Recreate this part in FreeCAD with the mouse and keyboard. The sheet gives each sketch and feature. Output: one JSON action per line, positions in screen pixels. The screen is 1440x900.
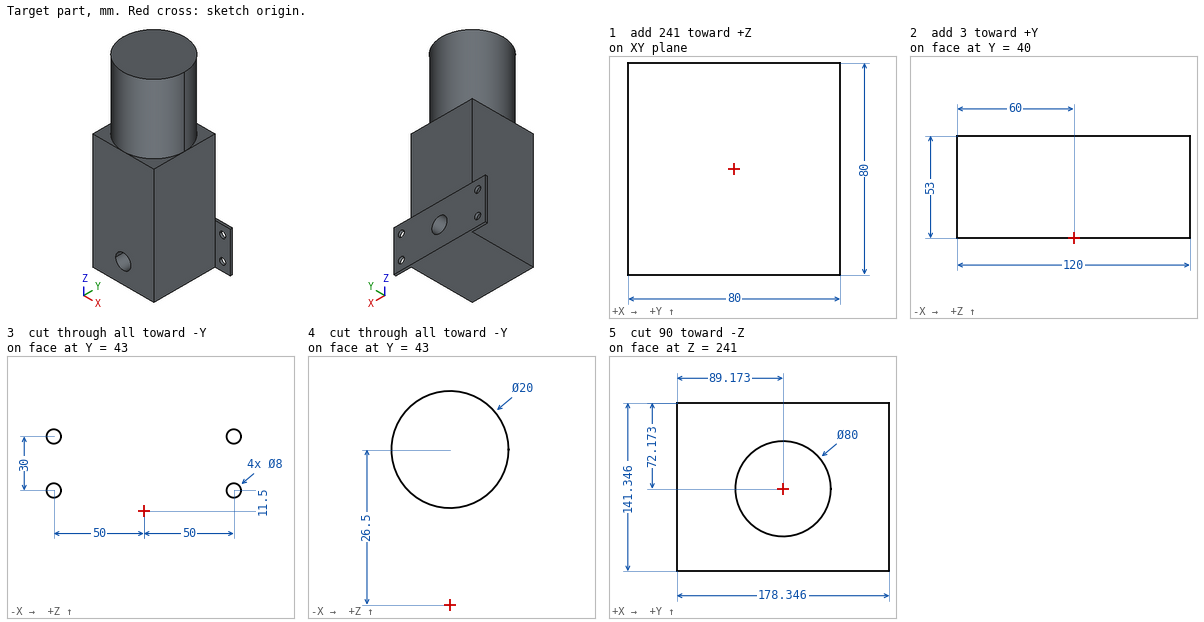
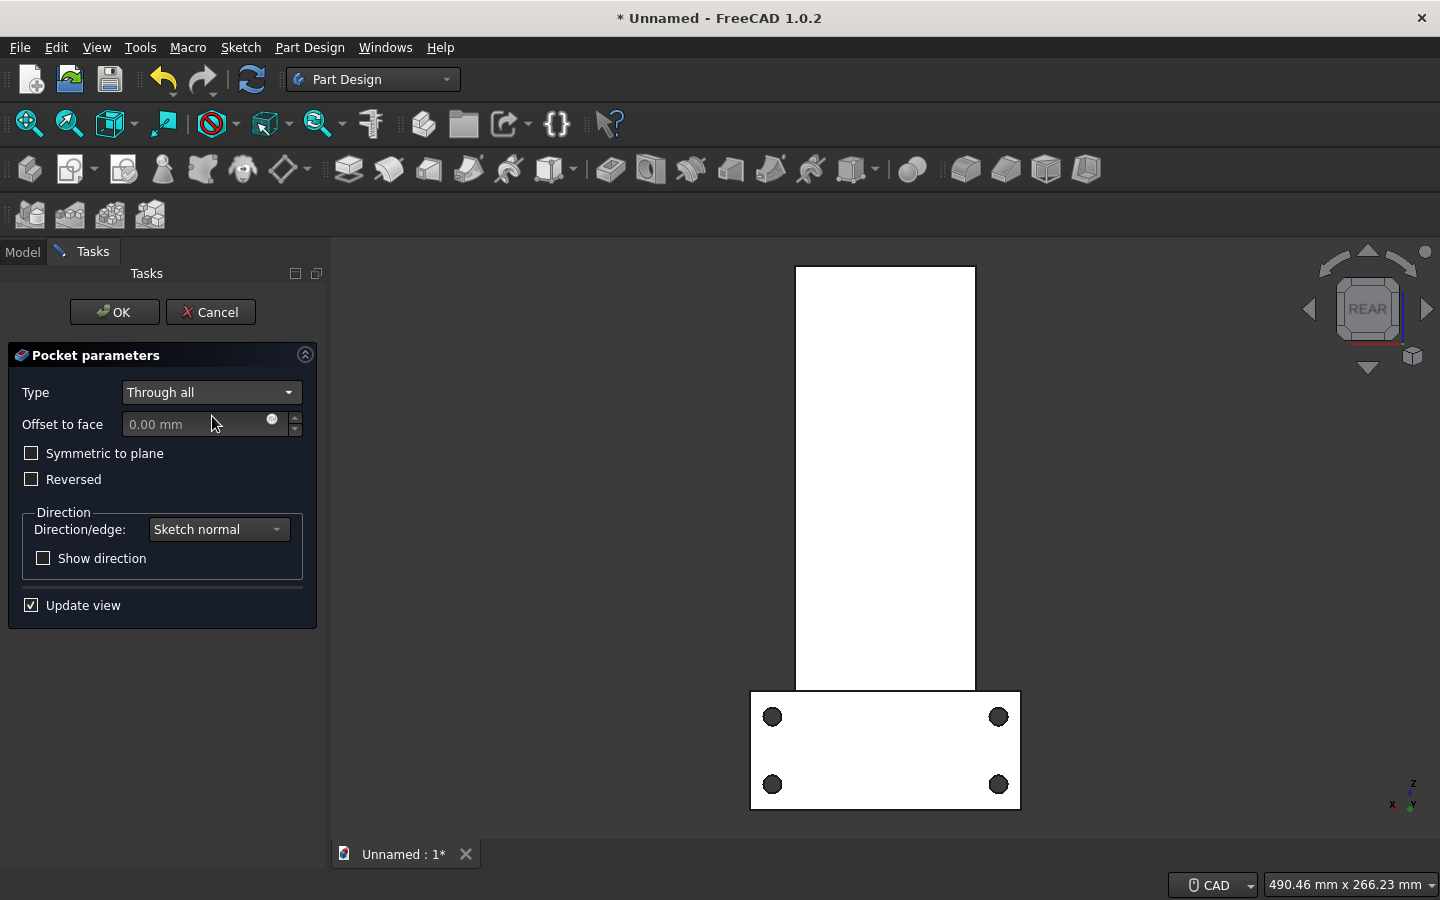
{"action": "left_click", "coordinate": [115, 312]}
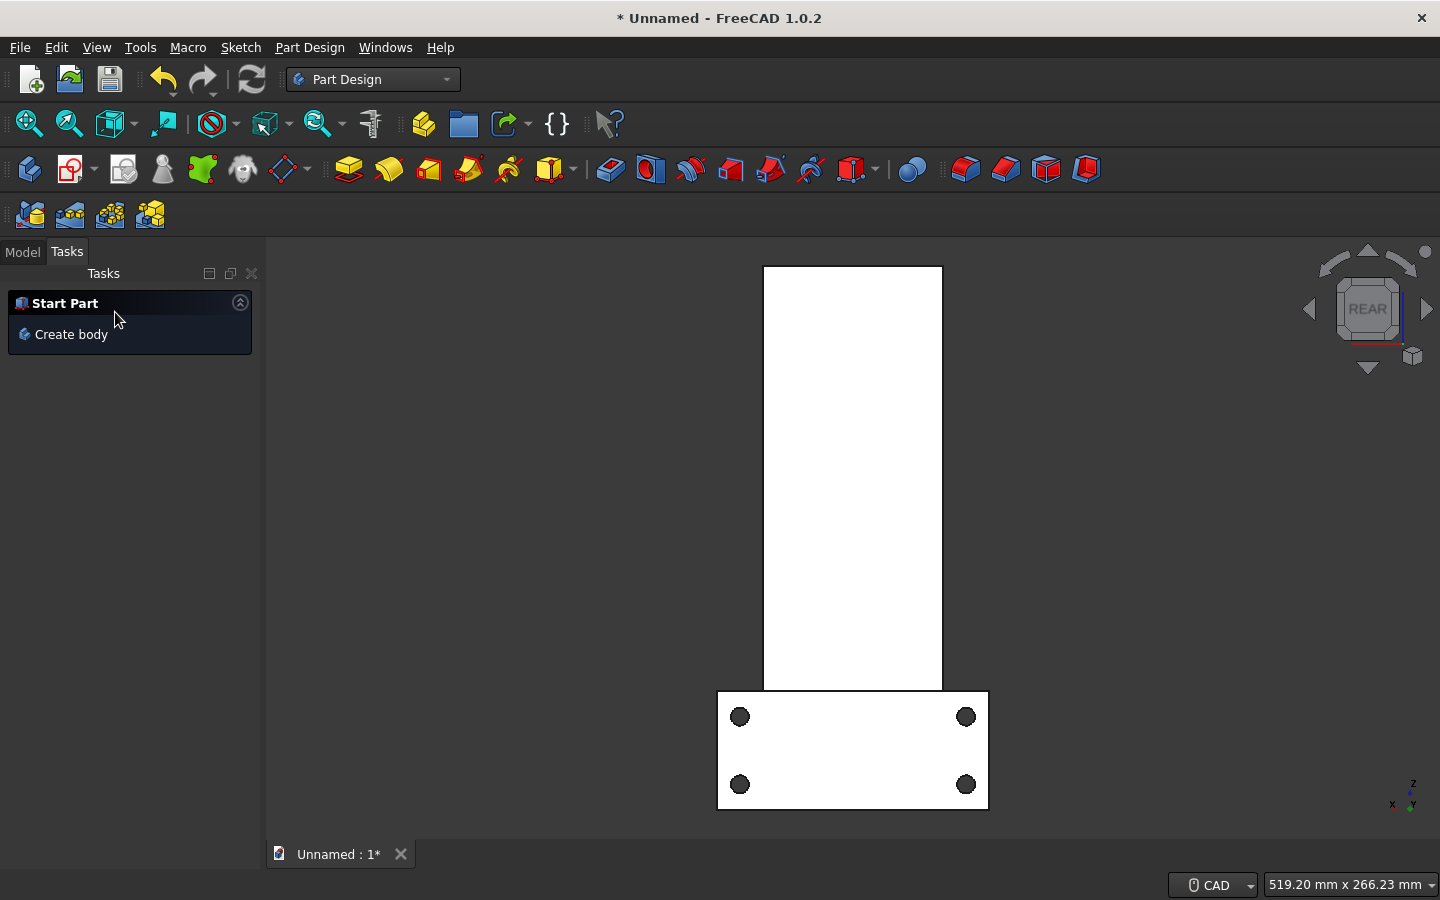
{"action": "left_click", "coordinate": [814, 750]}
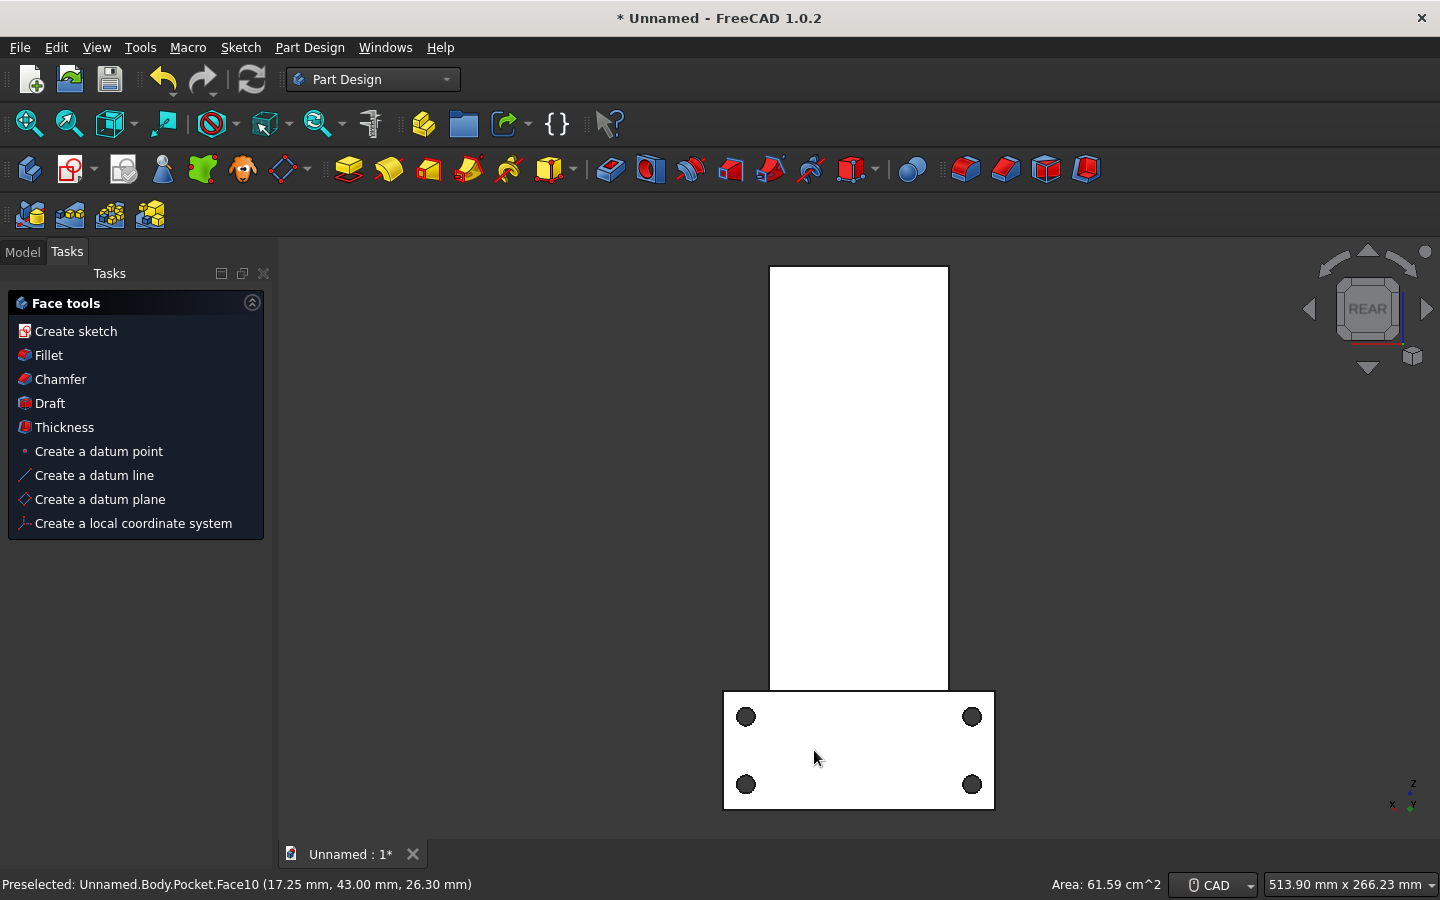
{"action": "left_click", "coordinate": [70, 170]}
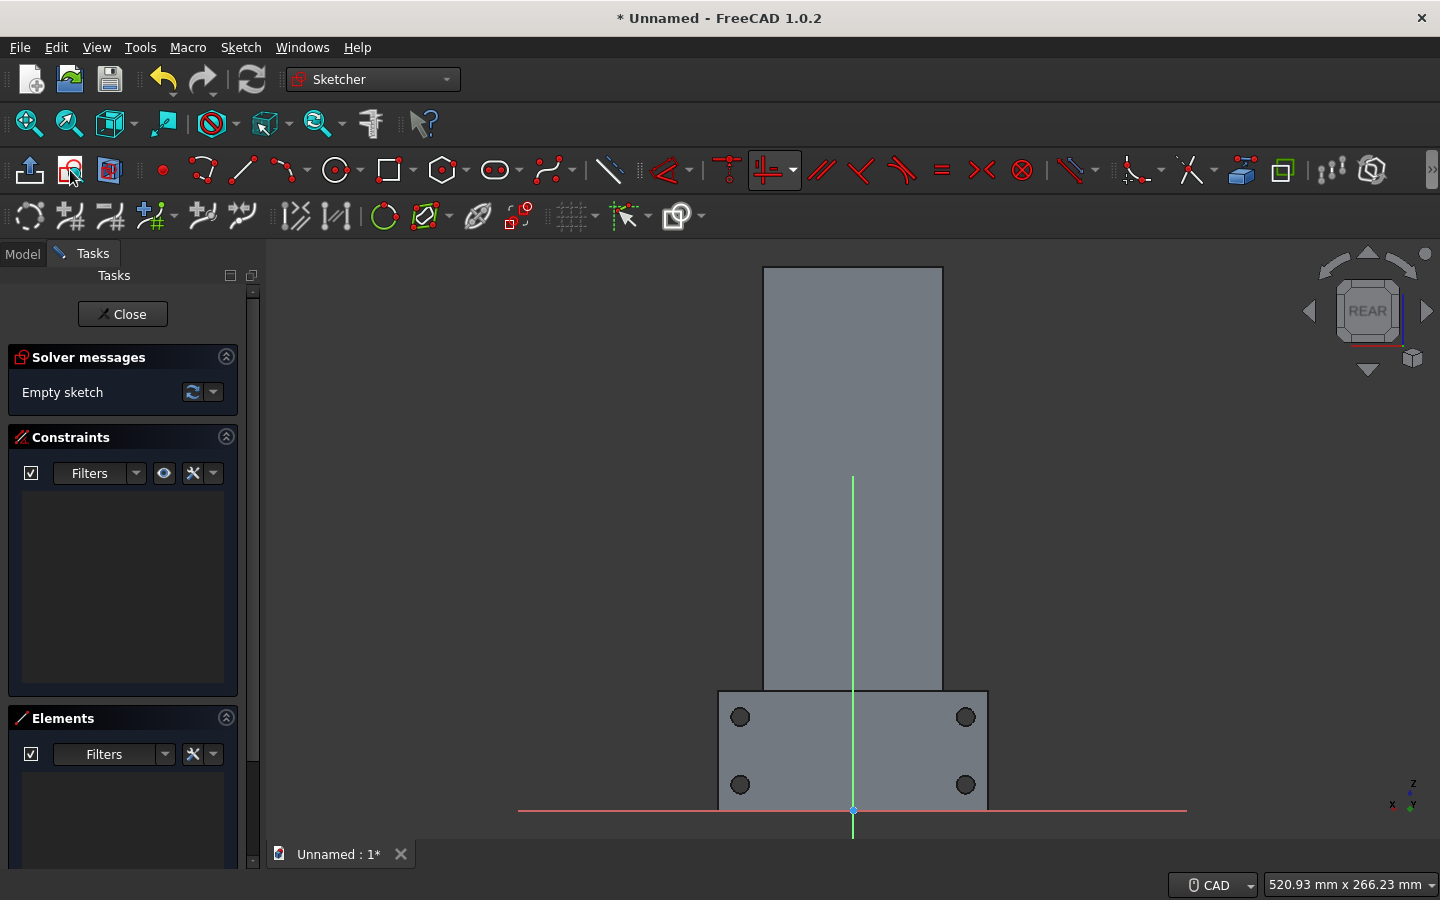
{"action": "scroll", "coordinate": [784, 539], "scroll_direction": "down", "scroll_amount": 5}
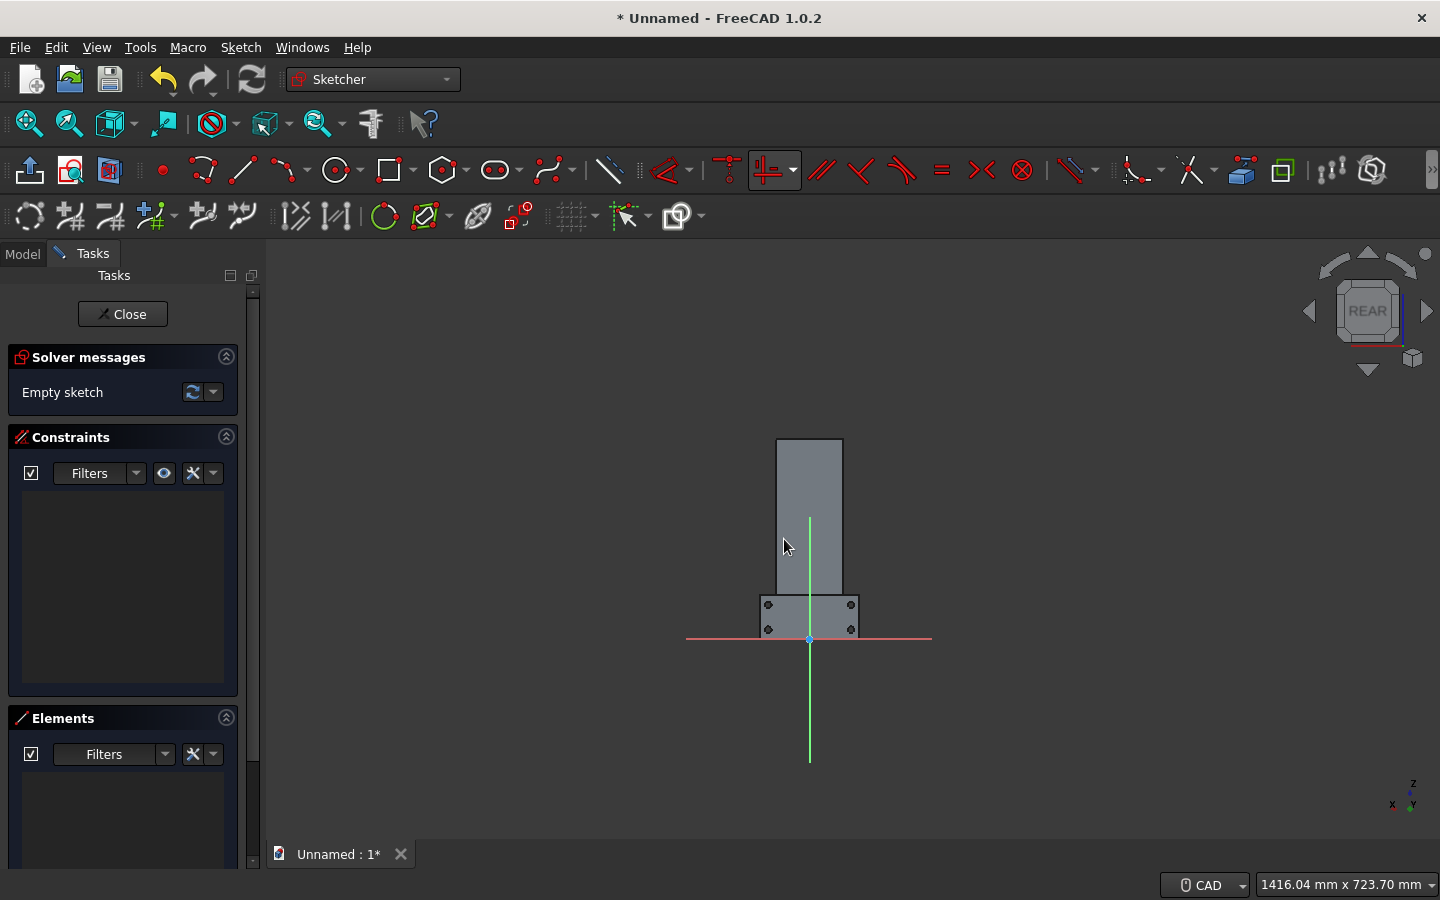
{"action": "scroll", "coordinate": [812, 631], "scroll_direction": "up", "scroll_amount": 13}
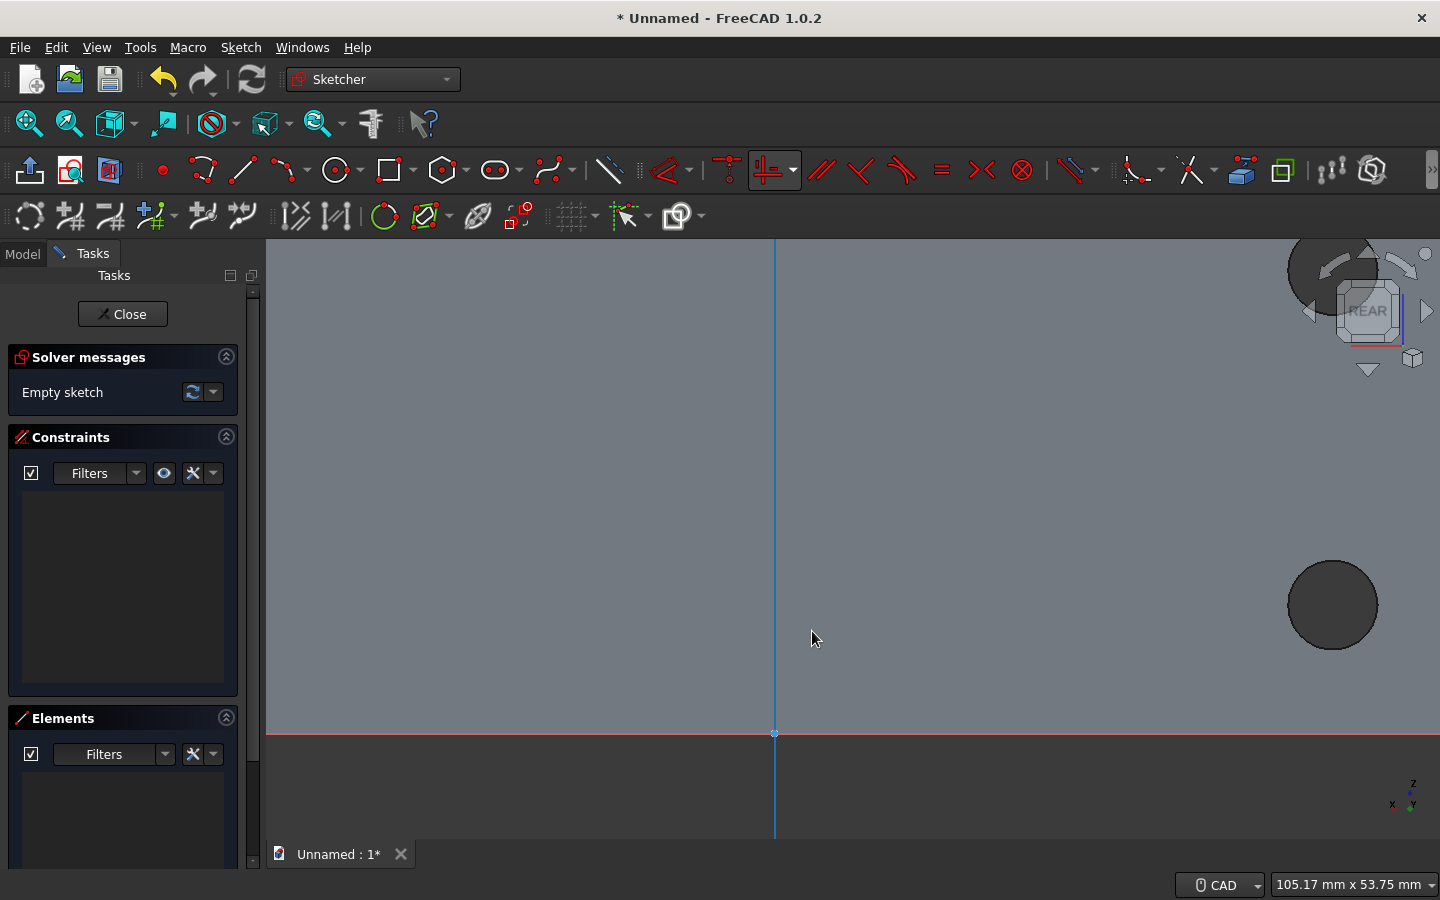
{"action": "left_click", "coordinate": [336, 170]}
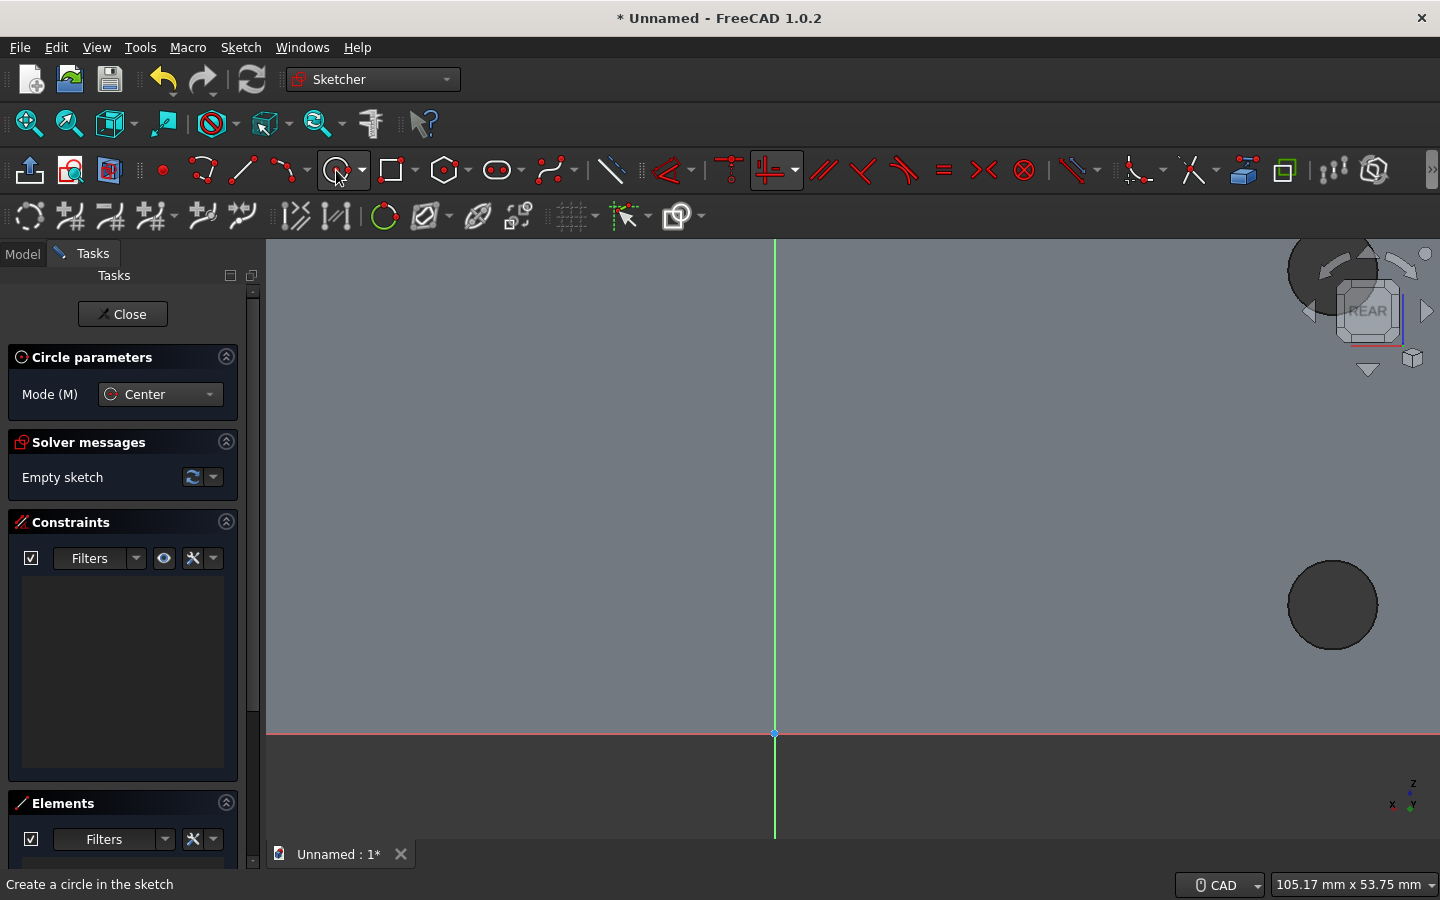
{"action": "left_click", "coordinate": [775, 438]}
{"action": "left_click", "coordinate": [854, 359]}
{"action": "key", "text": "Escape"}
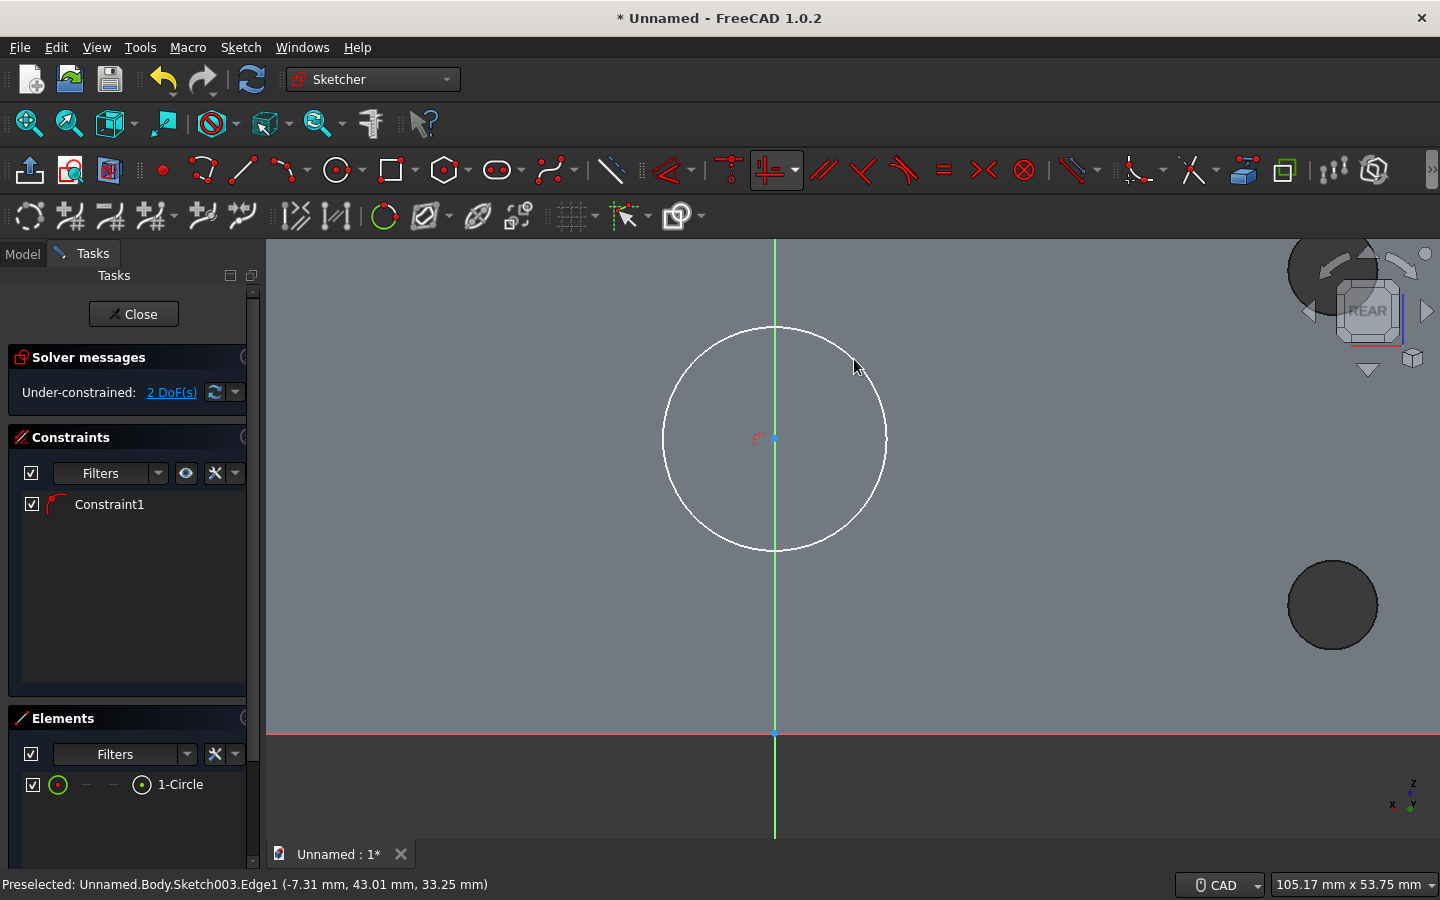
{"action": "key", "text": "d"}